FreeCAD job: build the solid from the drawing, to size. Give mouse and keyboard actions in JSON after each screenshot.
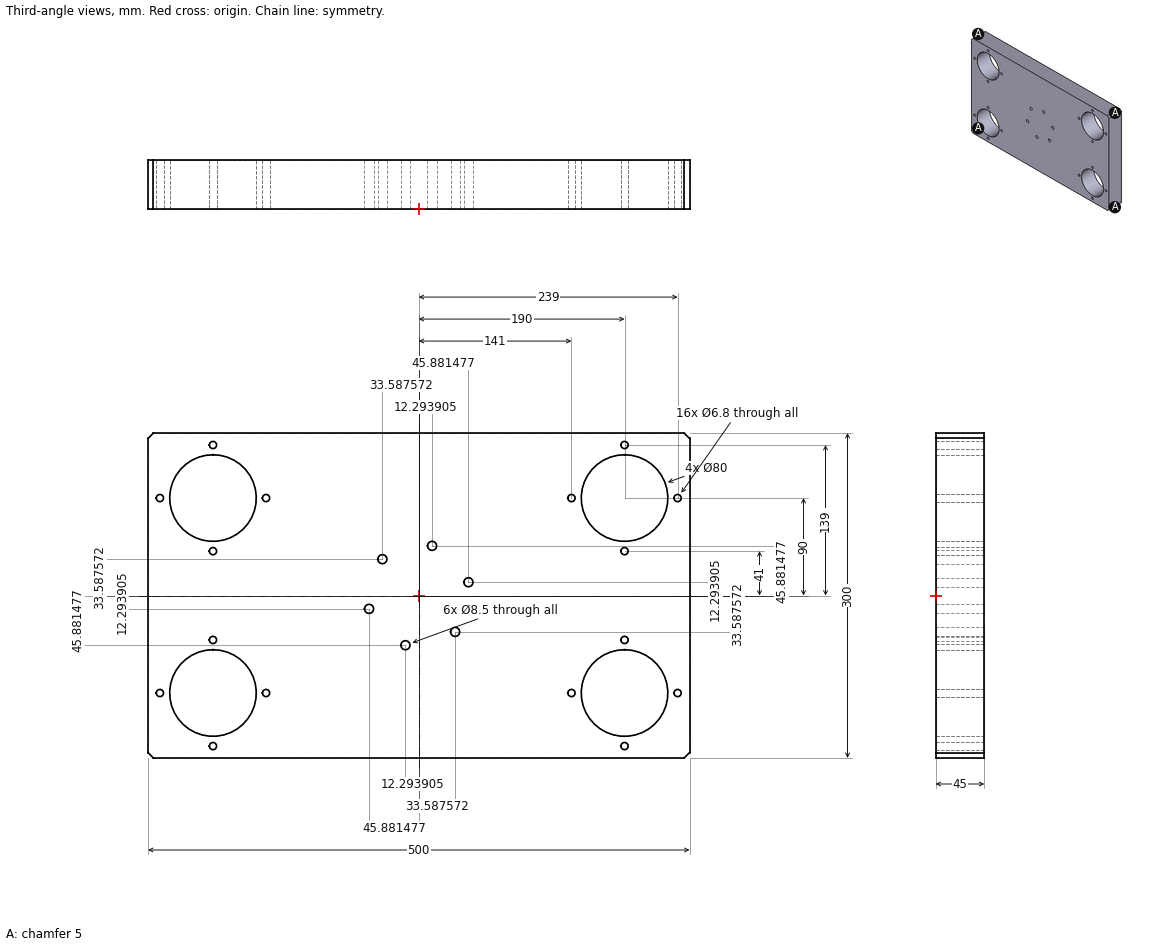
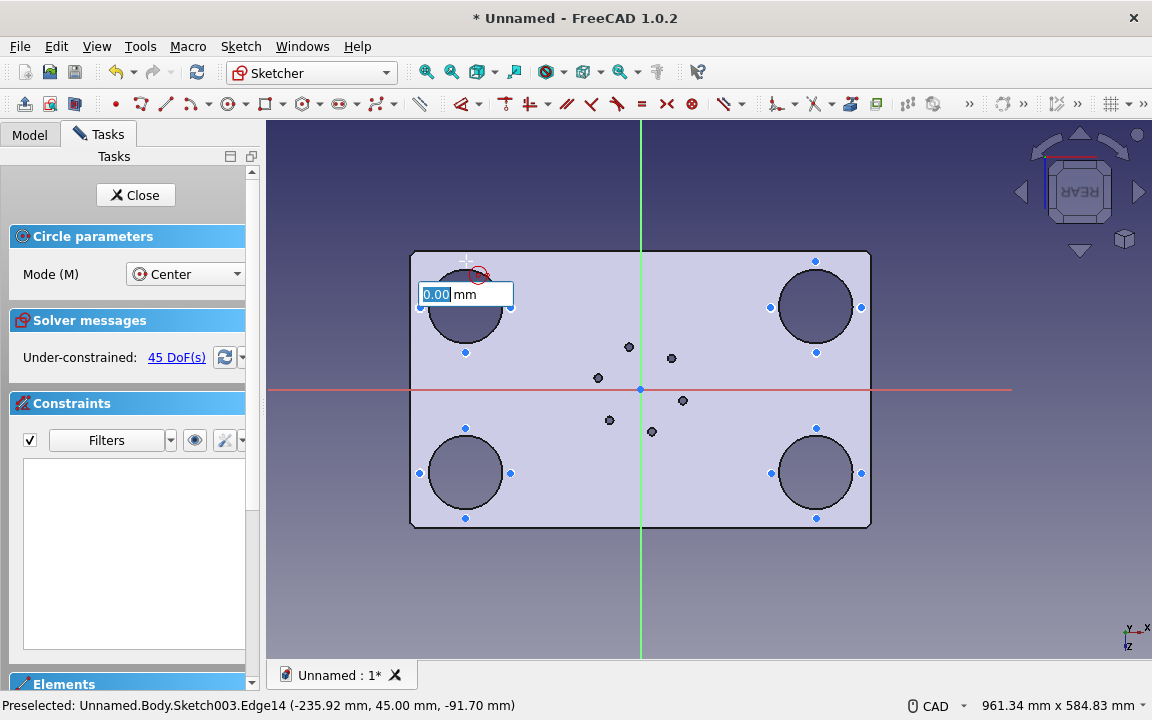
{"action": "scroll", "coordinate": [468, 259], "scroll_direction": "up", "scroll_amount": 9}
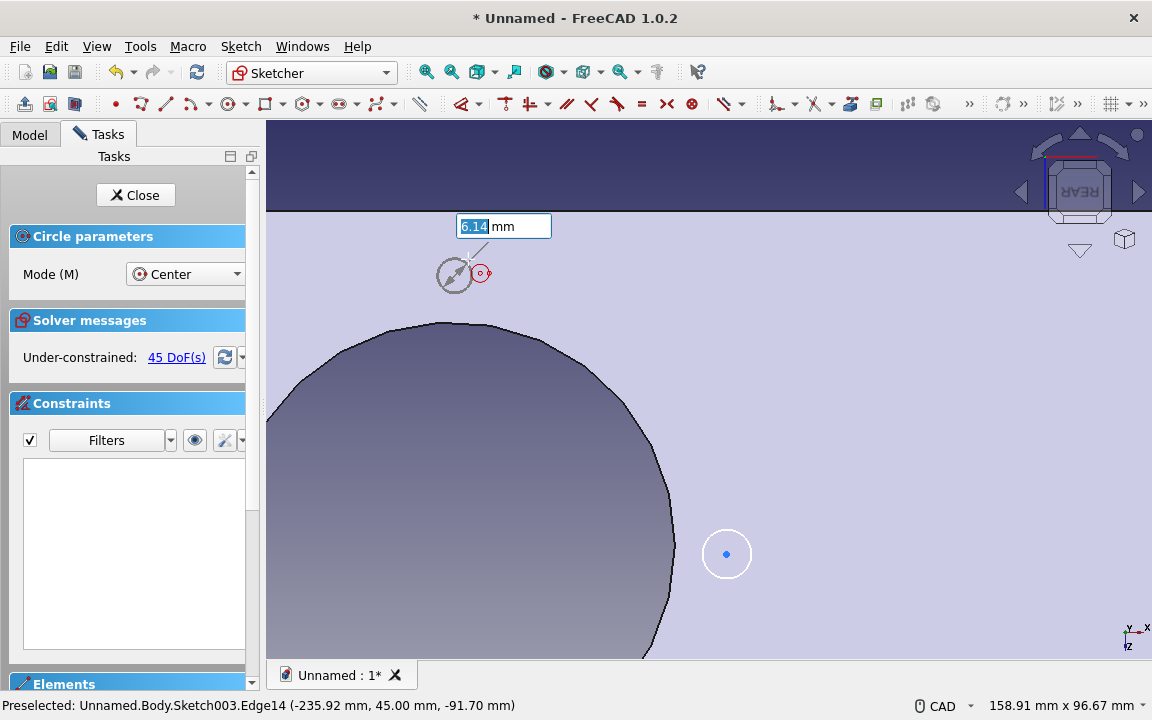
{"action": "left_click", "coordinate": [465, 259]}
{"action": "key", "text": "Escape"}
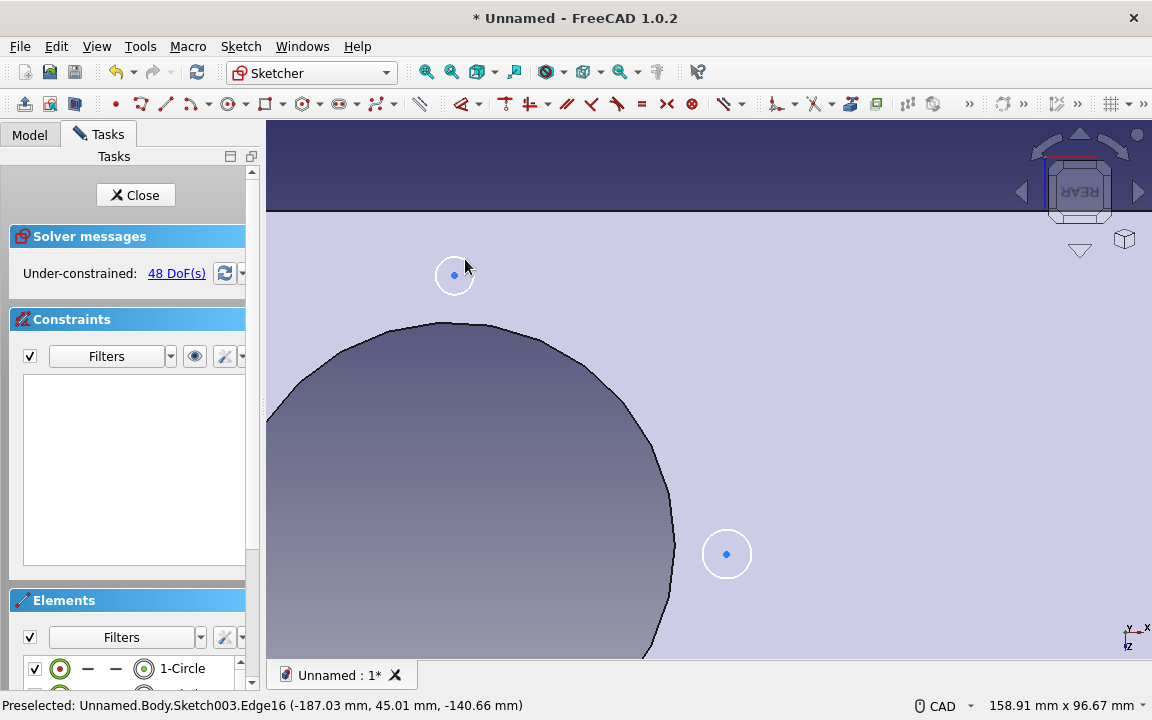
{"action": "scroll", "coordinate": [468, 259], "scroll_direction": "down", "scroll_amount": 9}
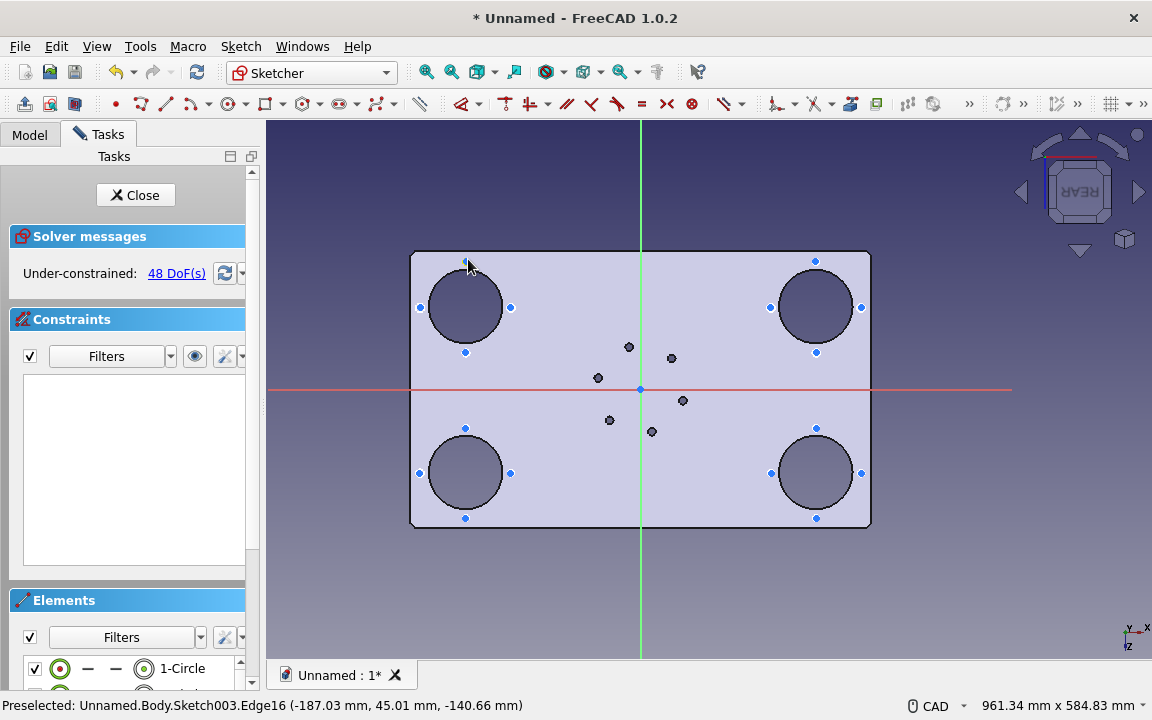
{"action": "scroll", "coordinate": [864, 471], "scroll_direction": "up", "scroll_amount": 8}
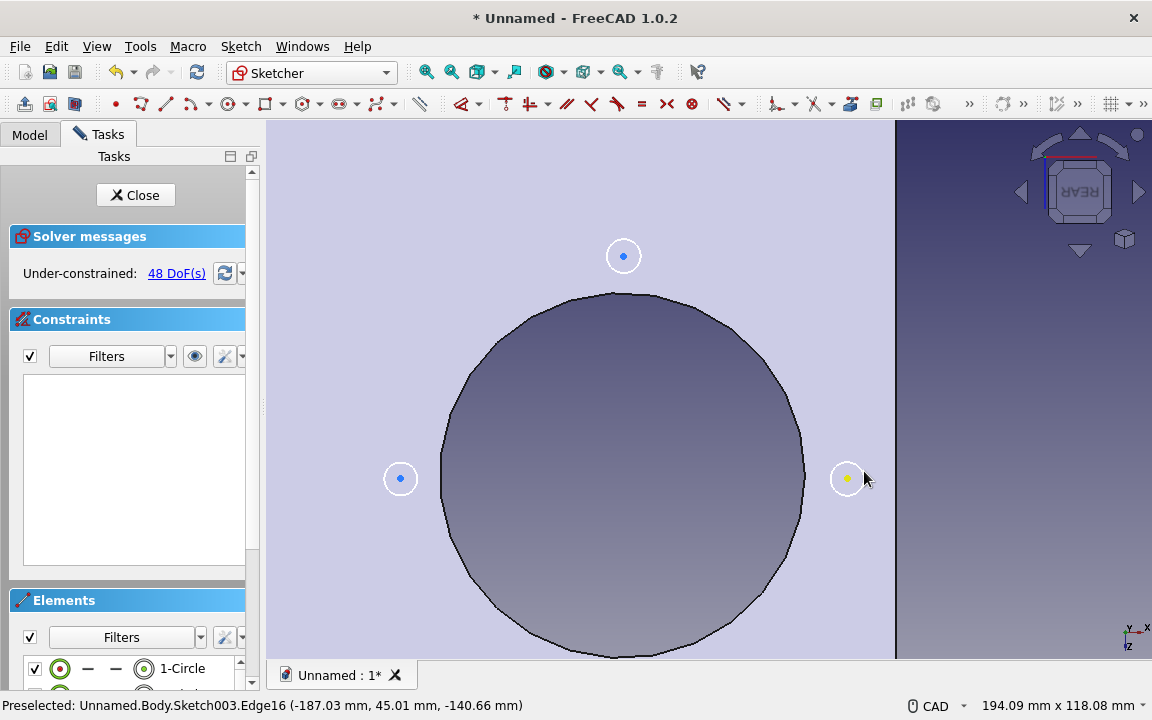
{"action": "left_click", "coordinate": [859, 467]}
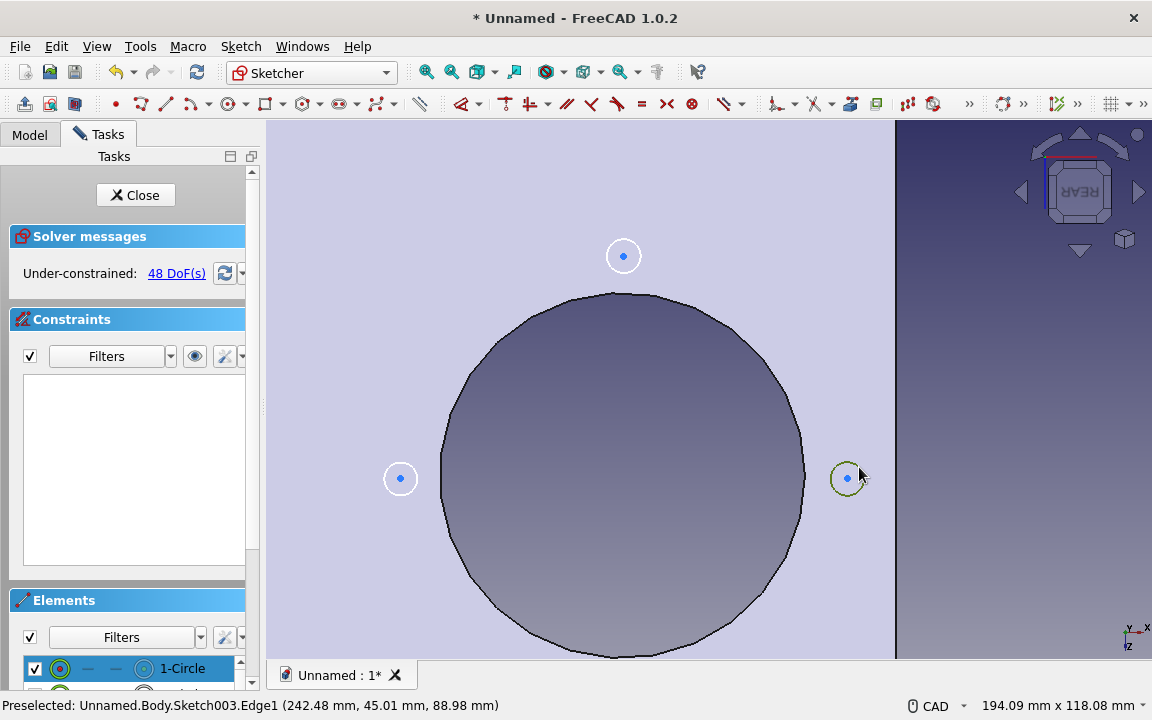
{"action": "scroll", "coordinate": [864, 472], "scroll_direction": "down", "scroll_amount": 8}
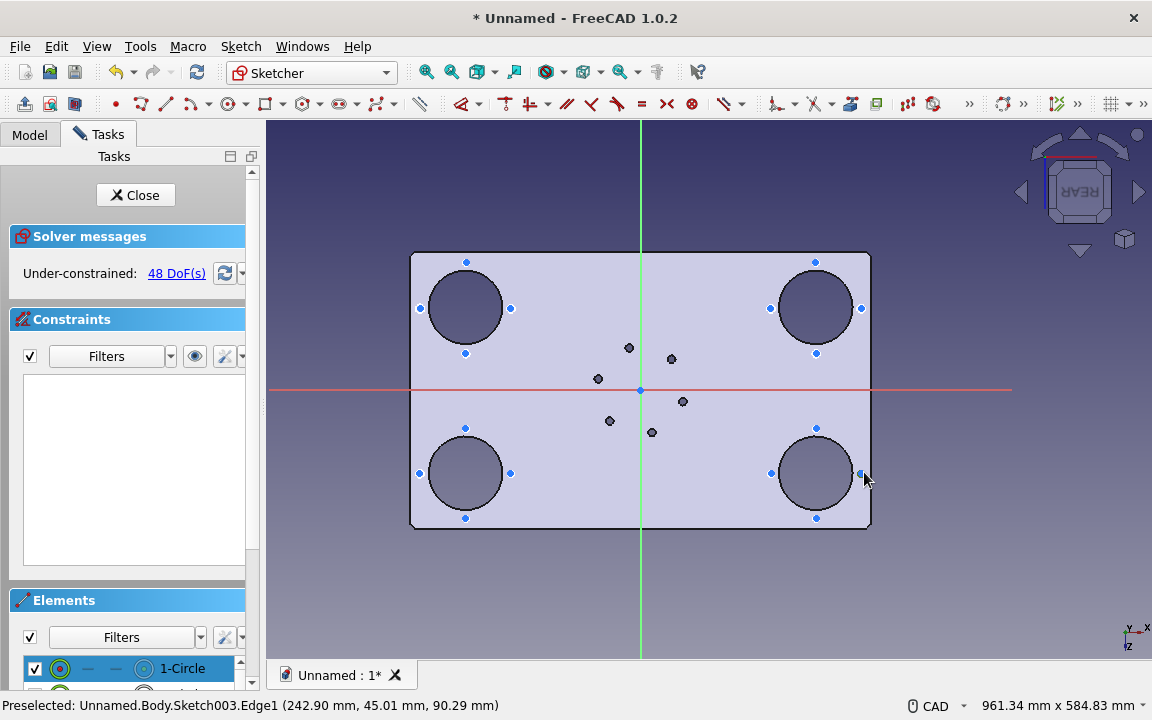
{"action": "scroll", "coordinate": [818, 517], "scroll_direction": "up", "scroll_amount": 8}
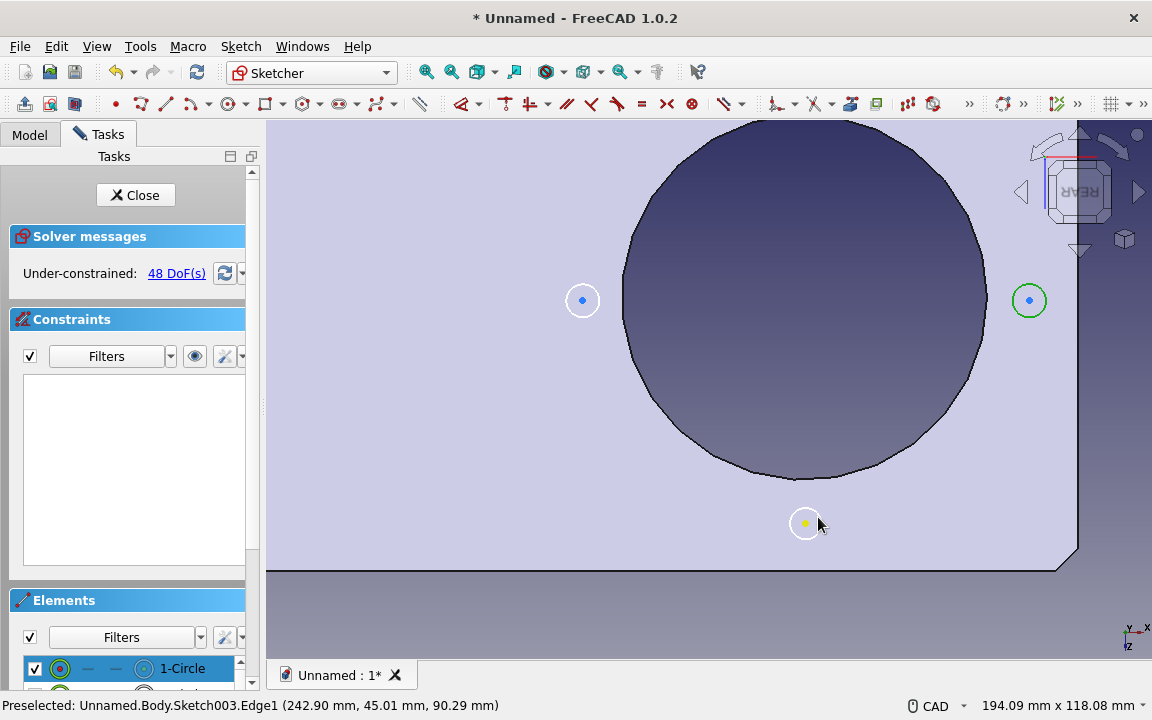
{"action": "left_click", "coordinate": [817, 513]}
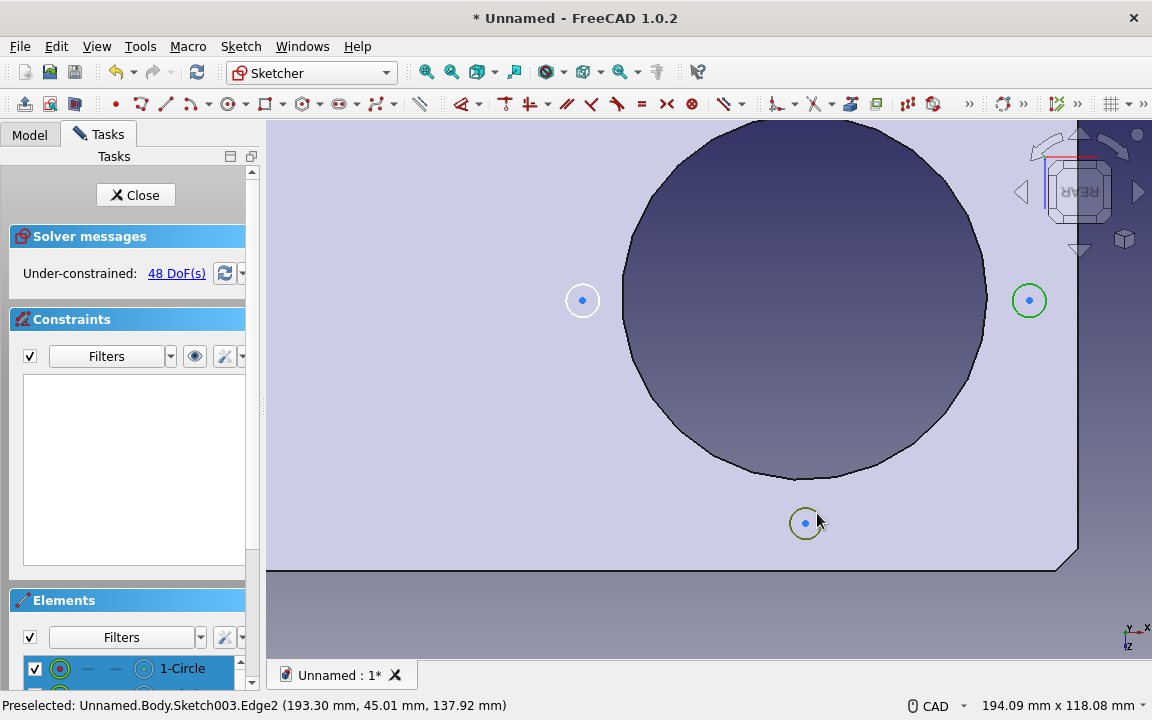
{"action": "left_click", "coordinate": [595, 289]}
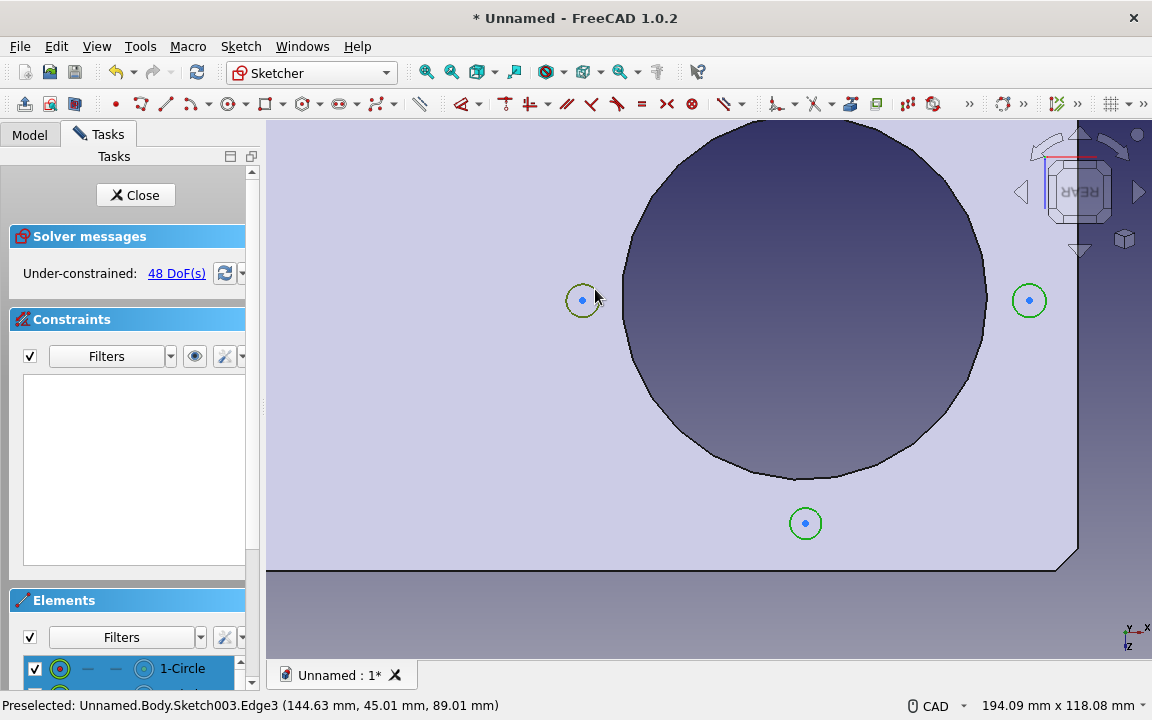
{"action": "scroll", "coordinate": [818, 517], "scroll_direction": "down", "scroll_amount": 8}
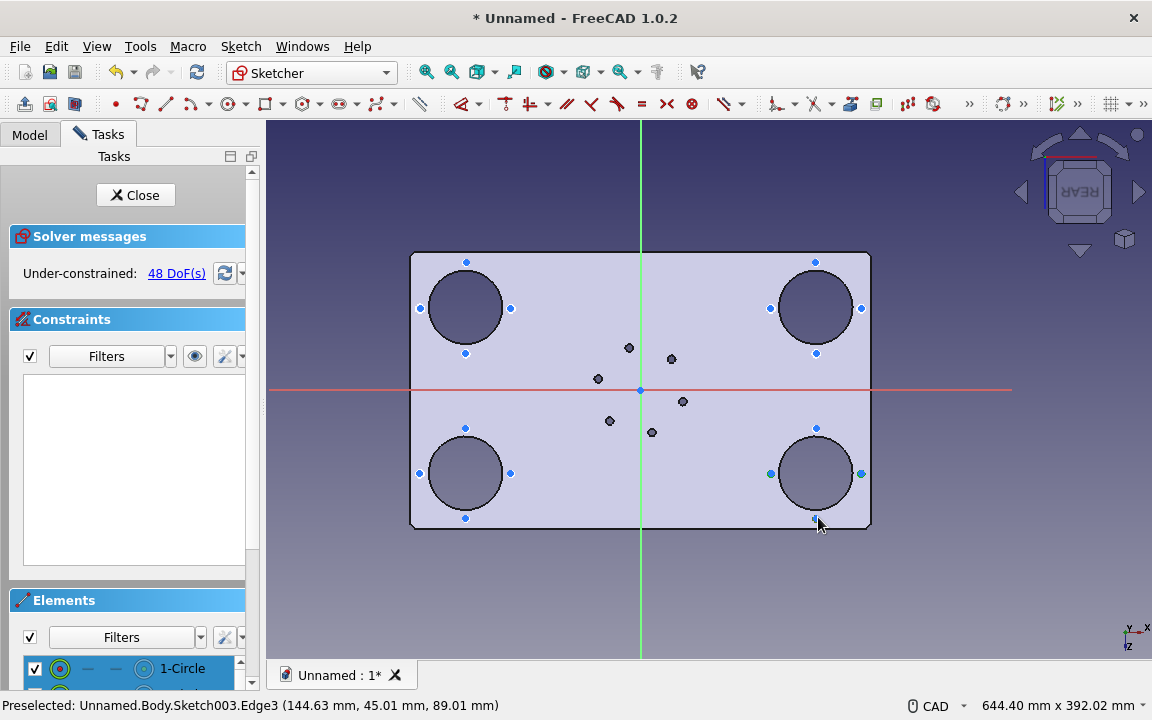
{"action": "scroll", "coordinate": [818, 427], "scroll_direction": "up", "scroll_amount": 7}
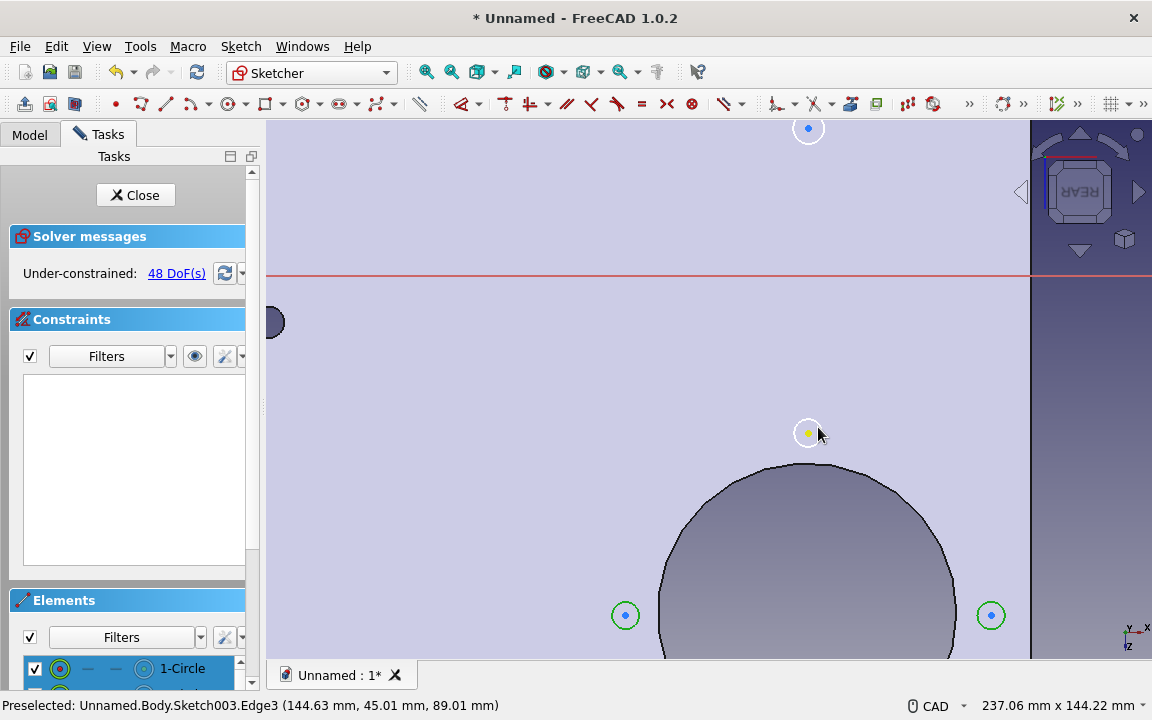
{"action": "left_click", "coordinate": [818, 423]}